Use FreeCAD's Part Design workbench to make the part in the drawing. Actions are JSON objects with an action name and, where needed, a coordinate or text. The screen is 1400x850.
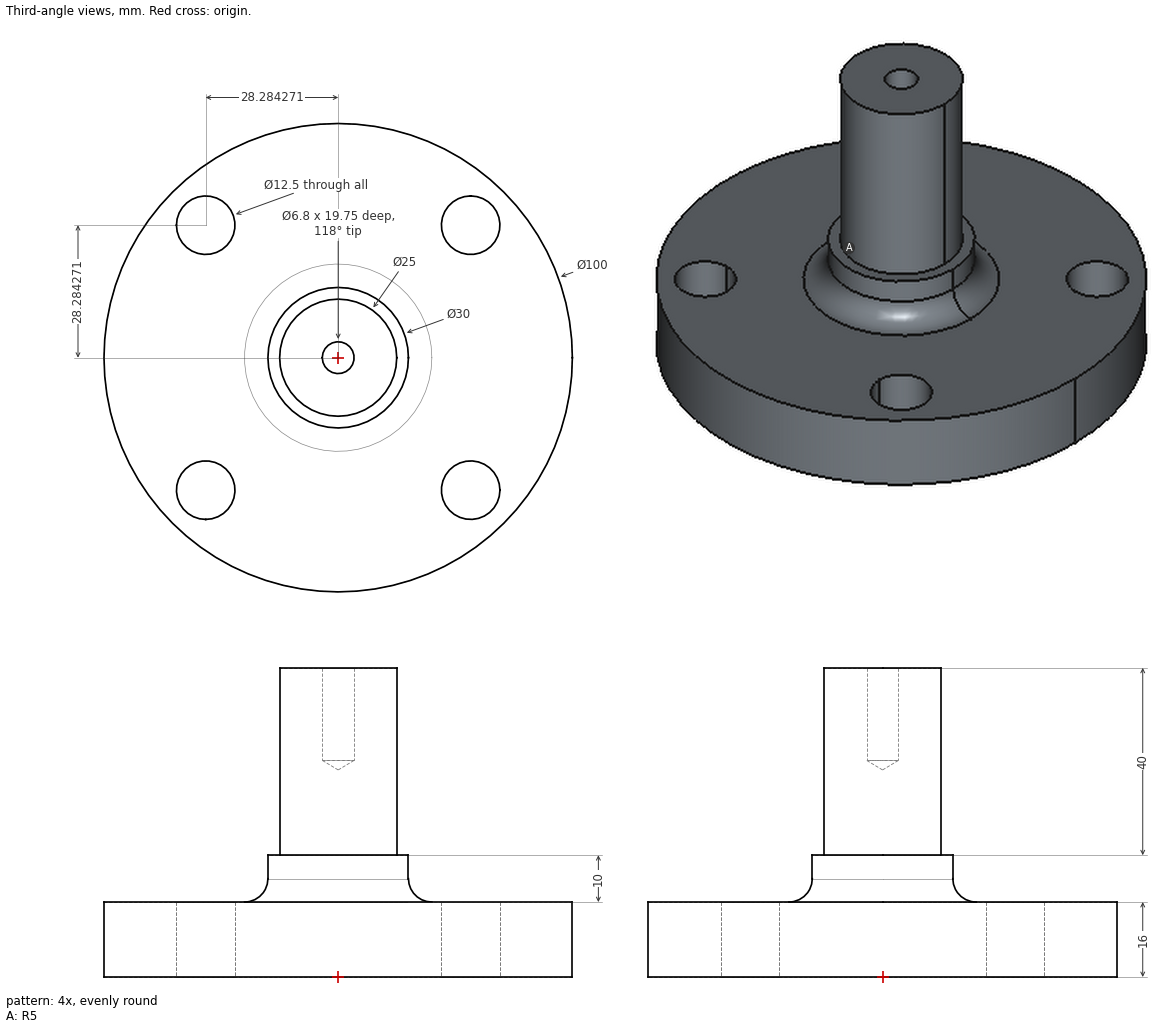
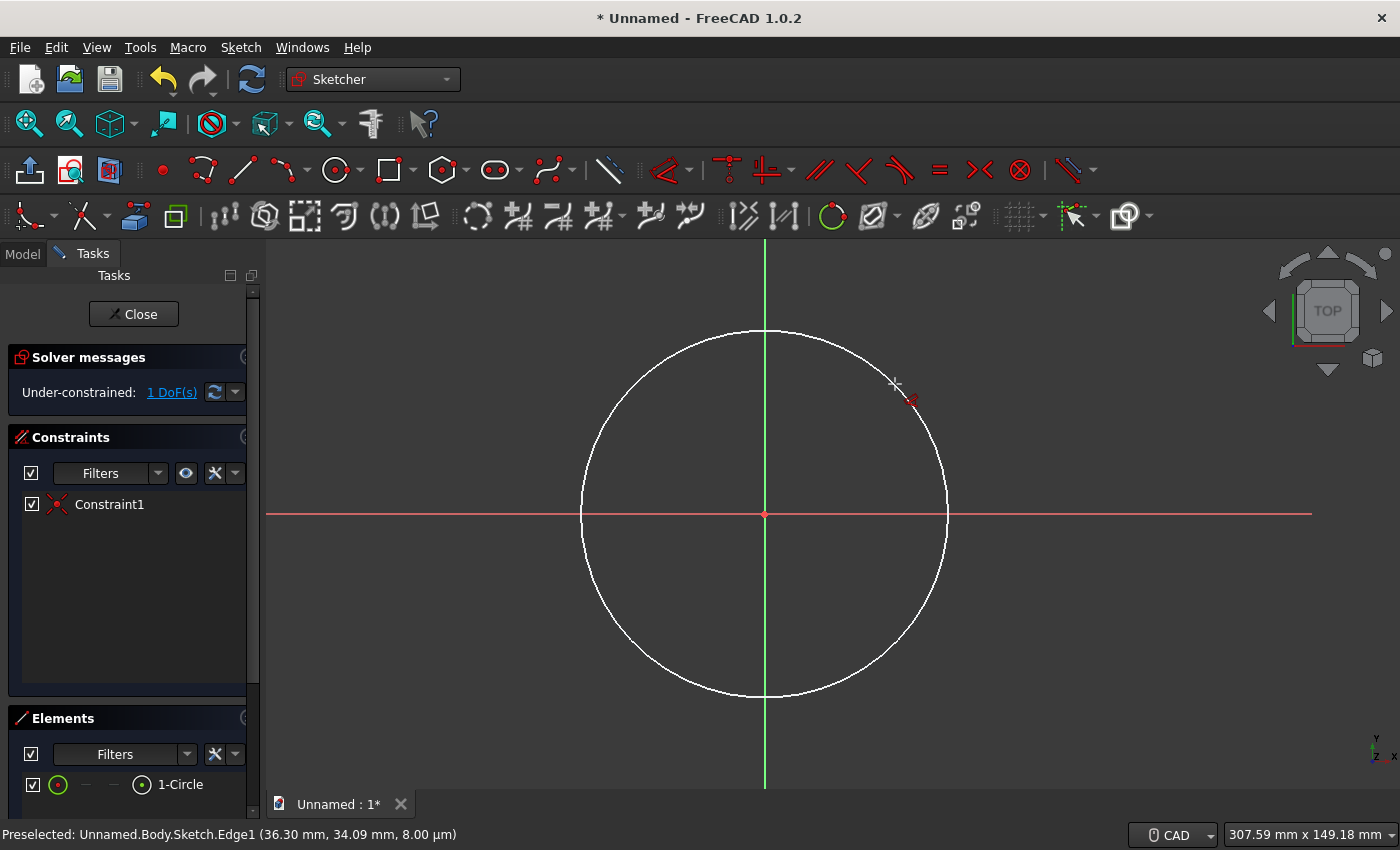
{"action": "left_click", "coordinate": [894, 384]}
{"action": "left_click", "coordinate": [917, 361]}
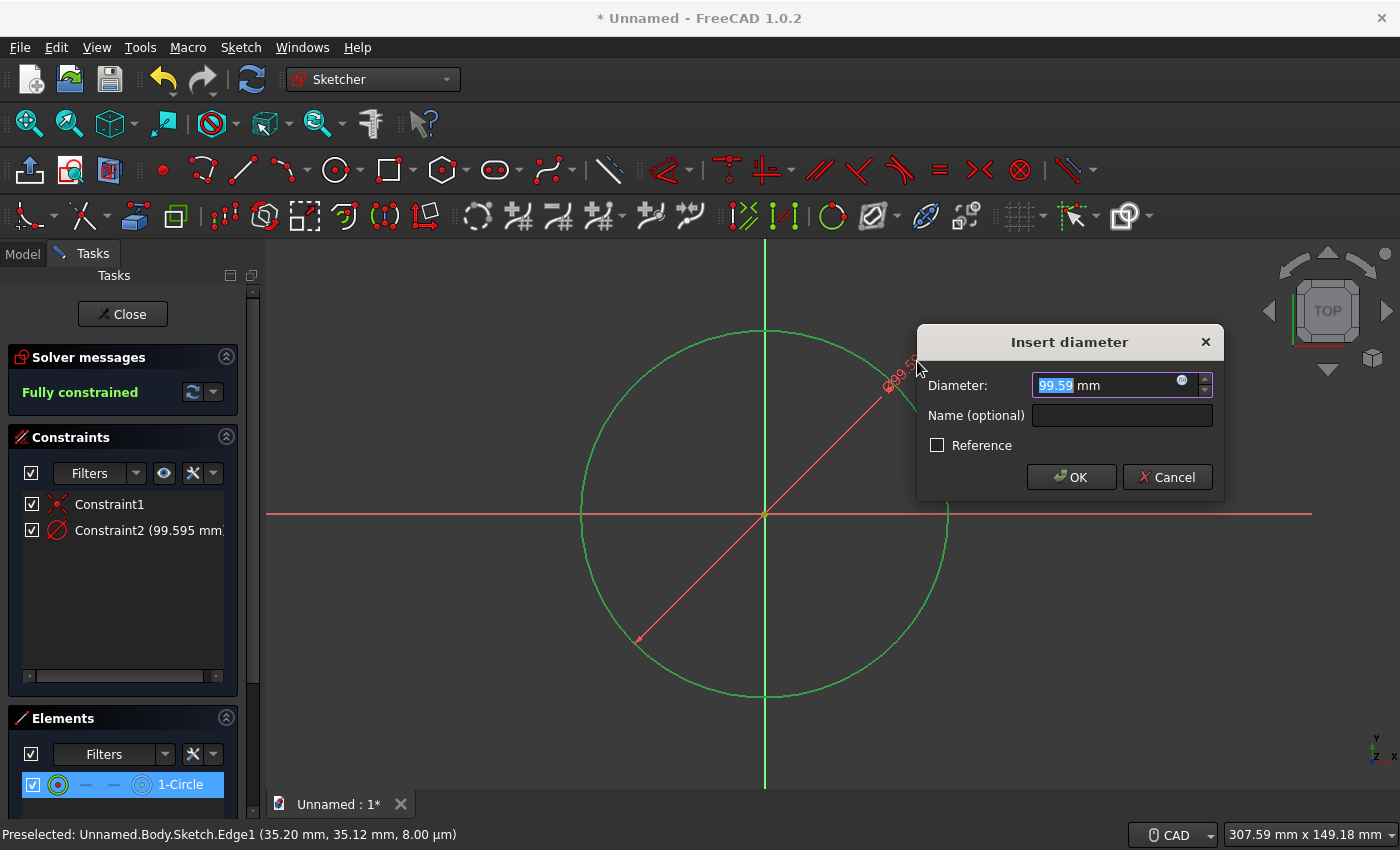
{"action": "type", "text": "100"}
{"action": "key", "text": "Return"}
{"action": "key", "text": "Escape"}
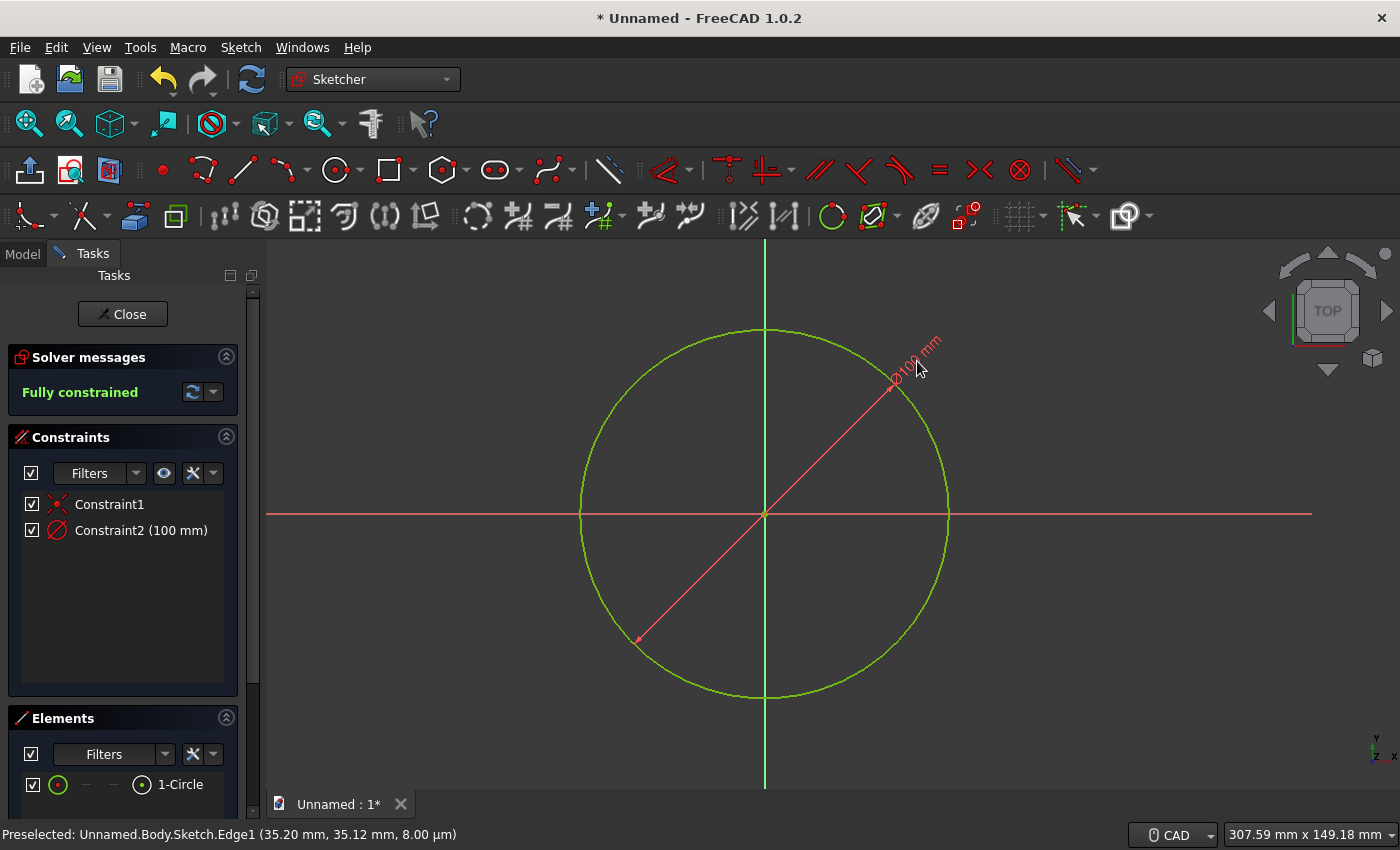
{"action": "left_click", "coordinate": [123, 314]}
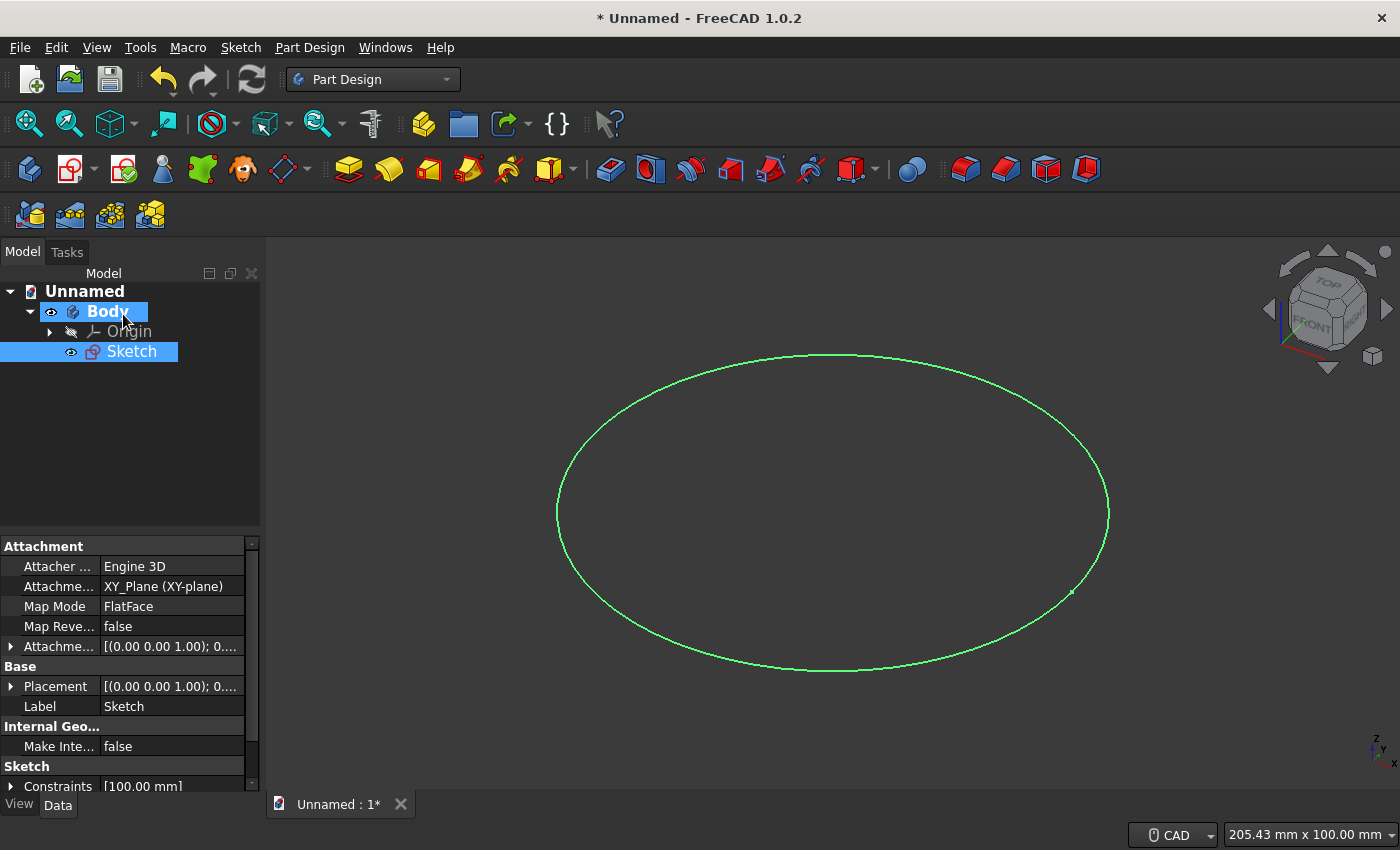
{"action": "left_click", "coordinate": [350, 170]}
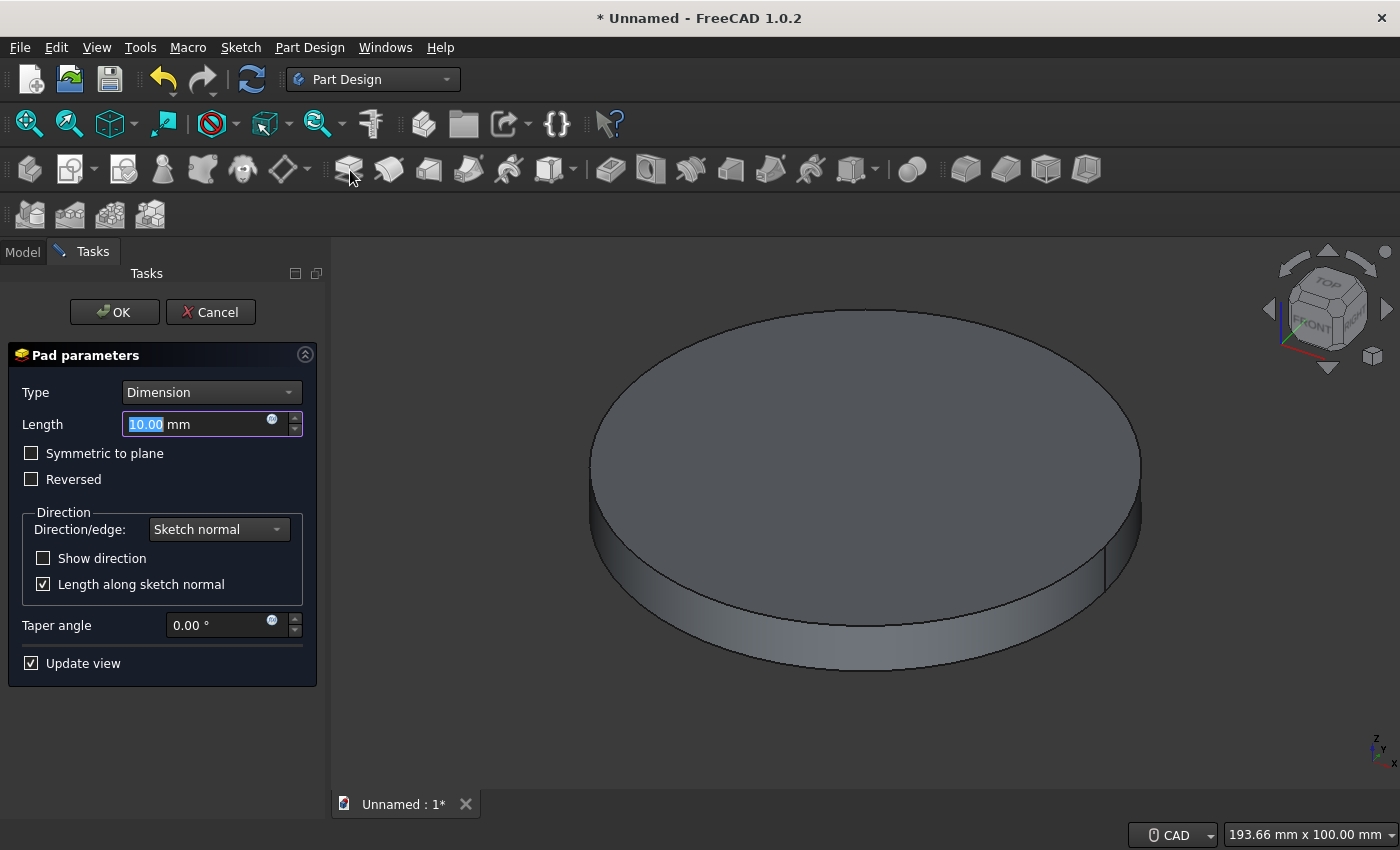
{"action": "type", "text": "16"}
{"action": "key", "text": "Tab"}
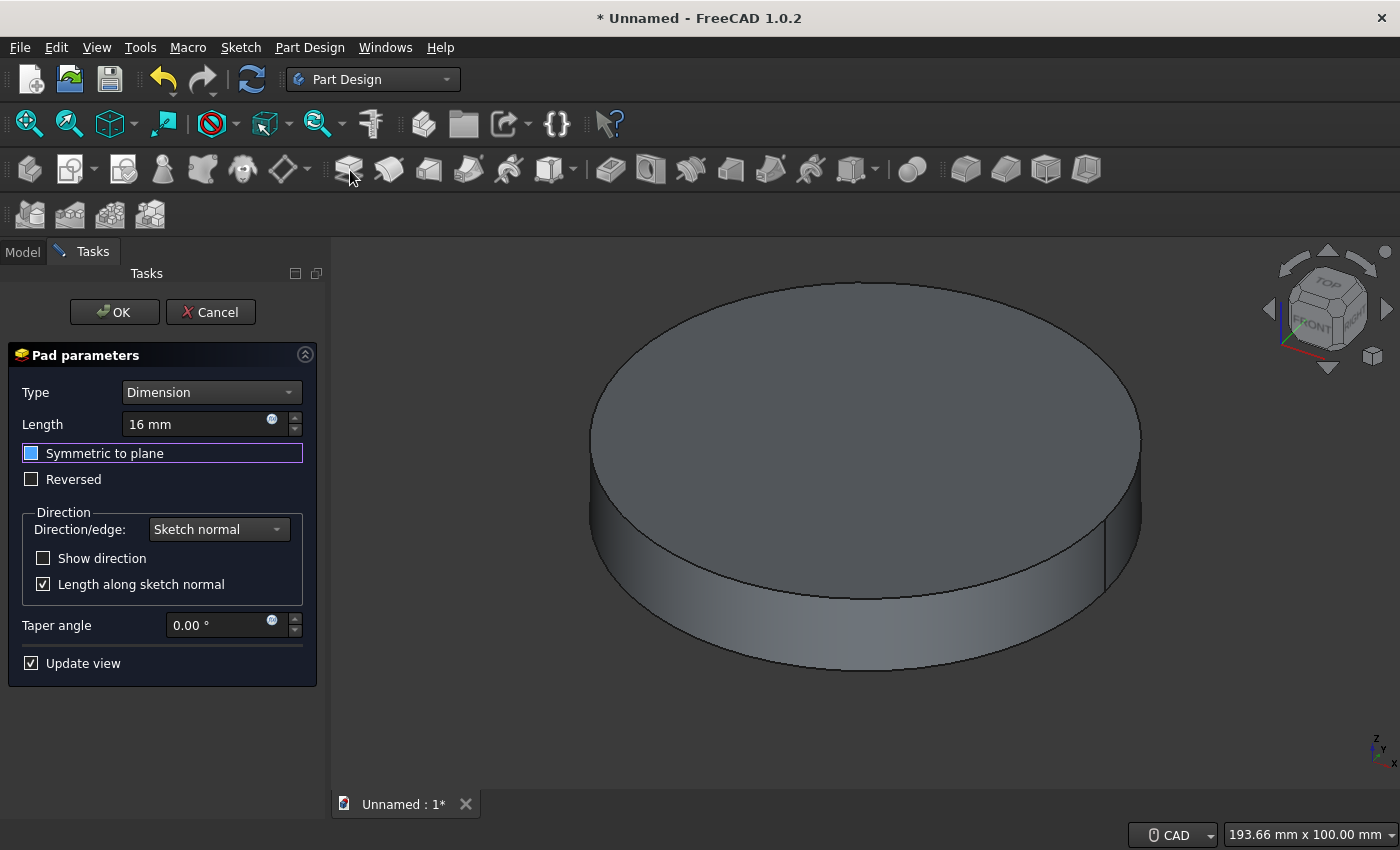
{"action": "left_click", "coordinate": [115, 312]}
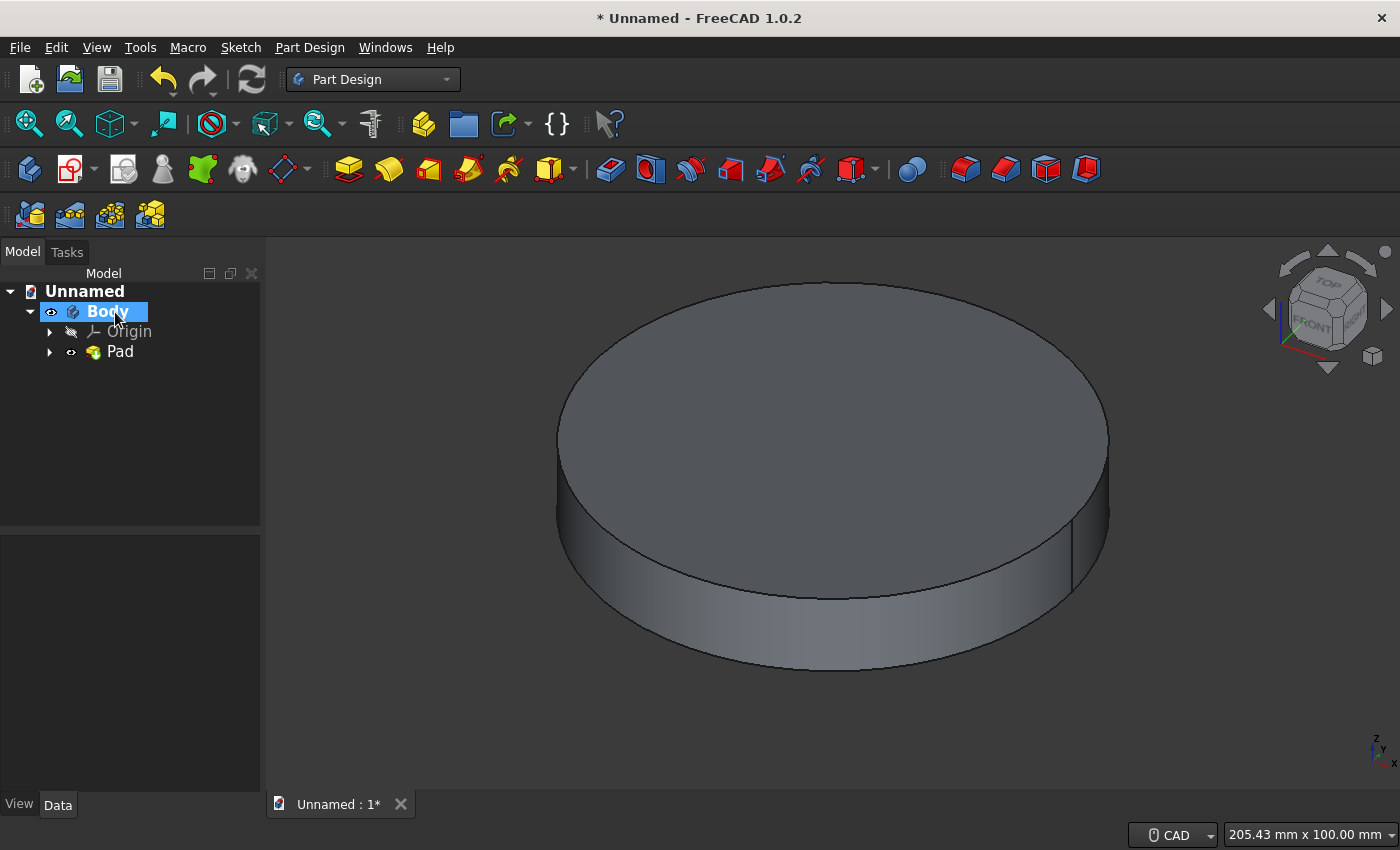
{"action": "key", "text": "v f"}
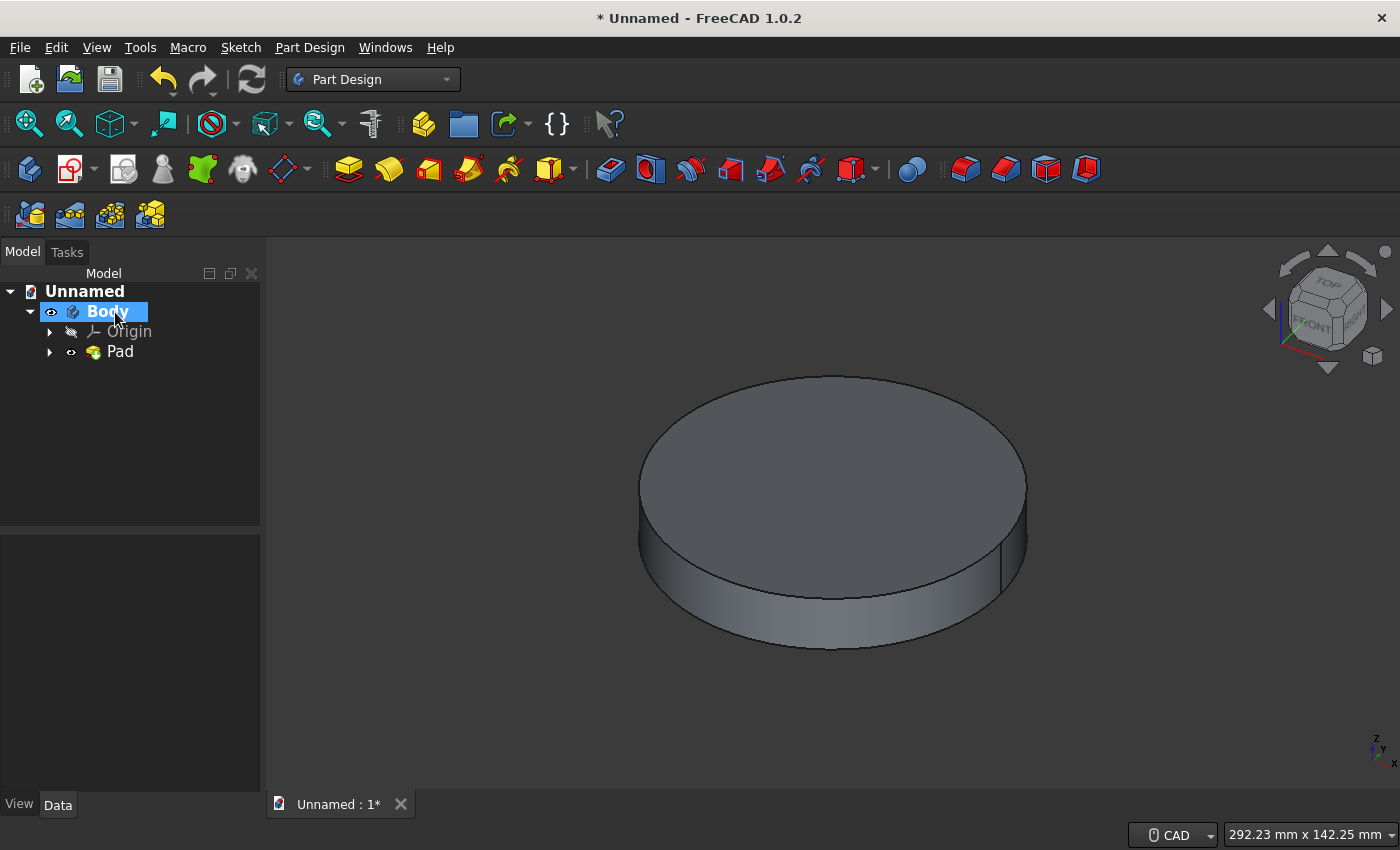
{"action": "left_click", "coordinate": [833, 487]}